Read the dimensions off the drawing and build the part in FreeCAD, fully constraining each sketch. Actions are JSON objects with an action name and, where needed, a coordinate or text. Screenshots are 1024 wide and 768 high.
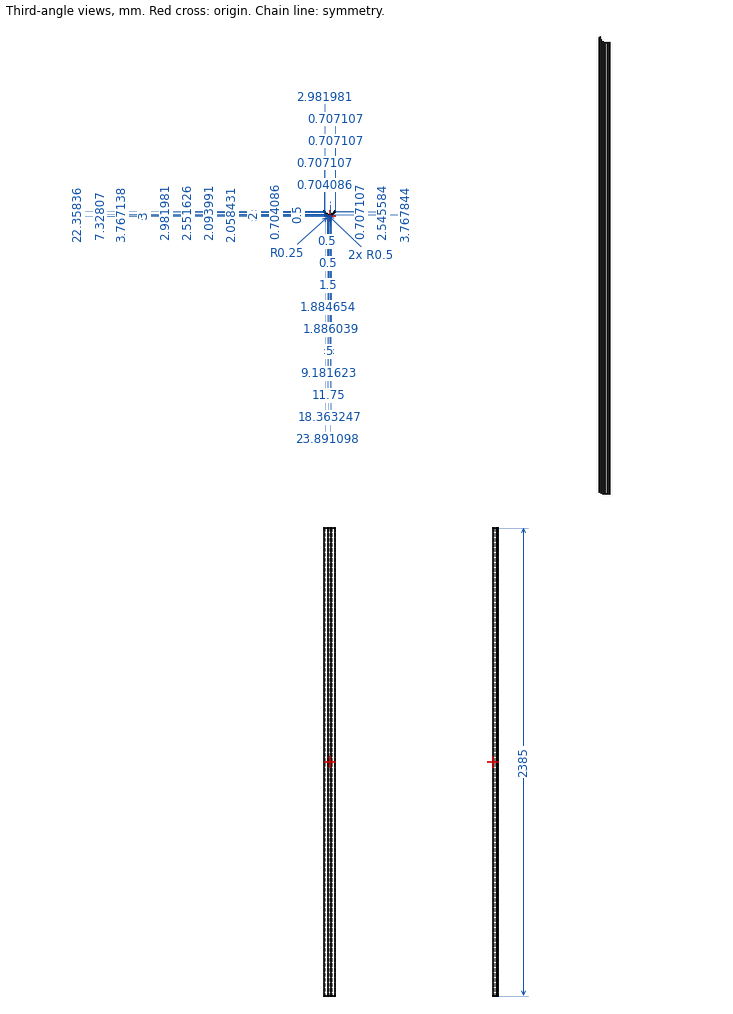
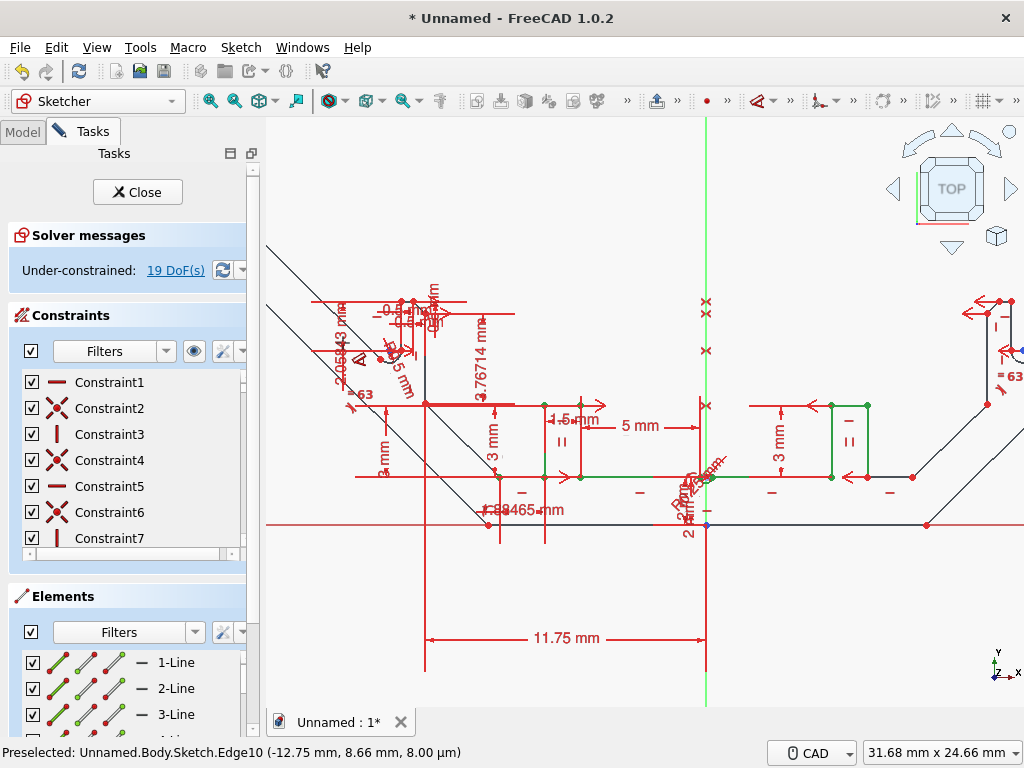
{"action": "scroll", "coordinate": [521, 478], "scroll_direction": "down", "scroll_amount": 6}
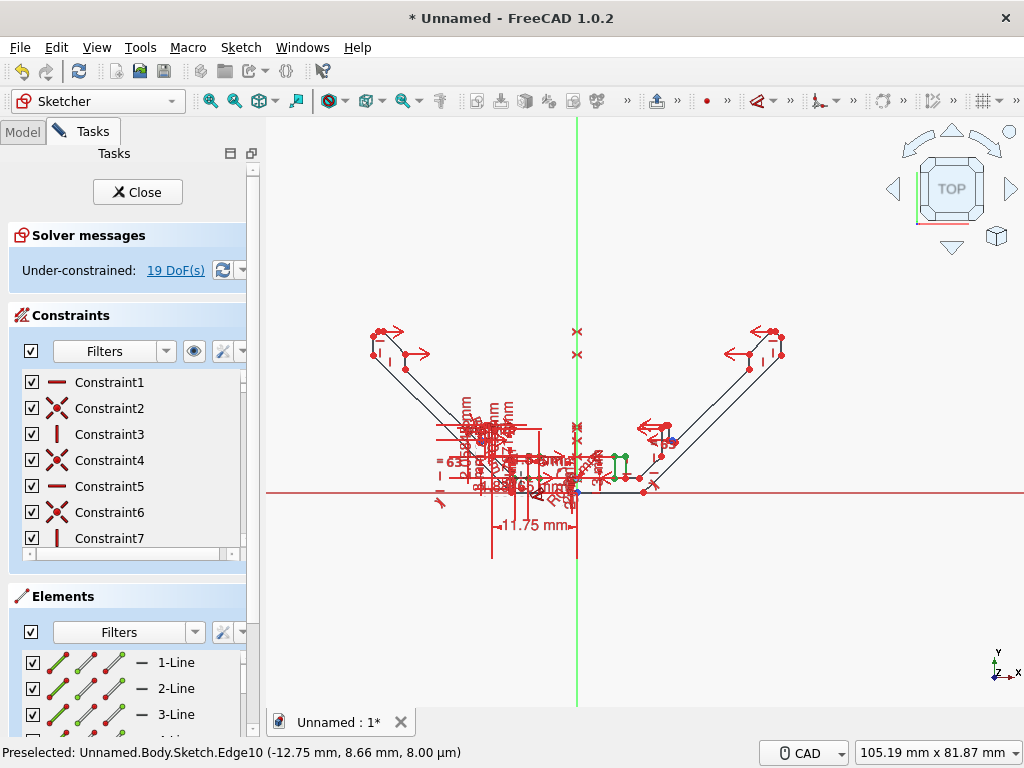
{"action": "scroll", "coordinate": [405, 365], "scroll_direction": "up", "scroll_amount": 6}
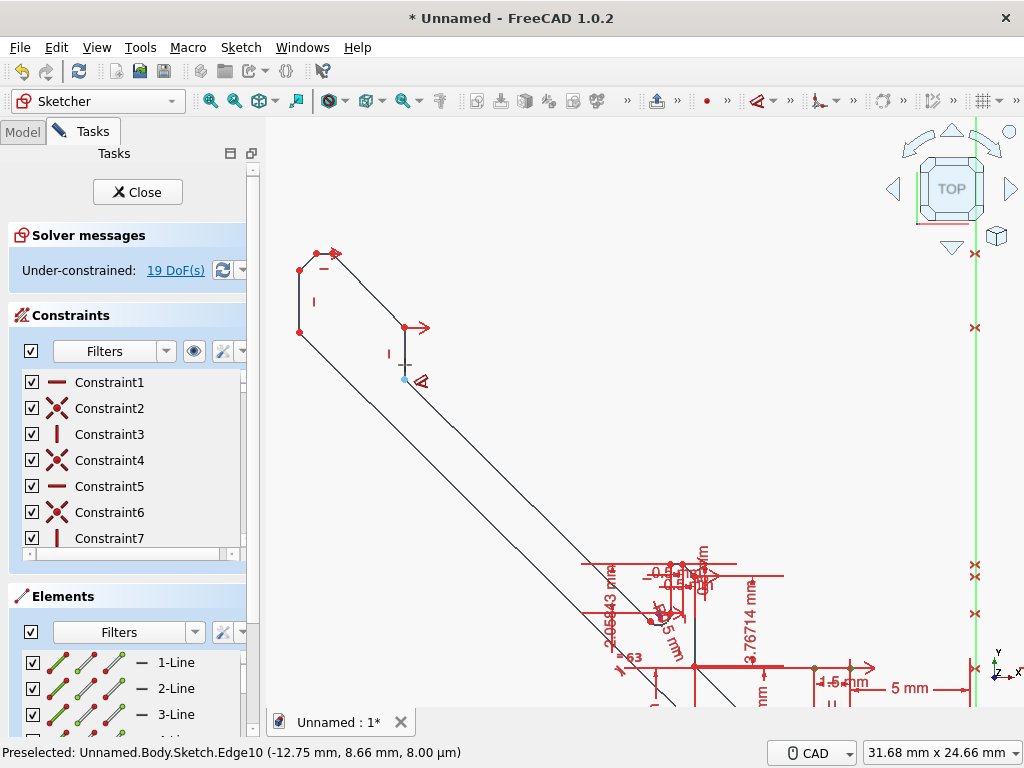
{"action": "left_click", "coordinate": [405, 364]}
{"action": "left_click", "coordinate": [371, 354]}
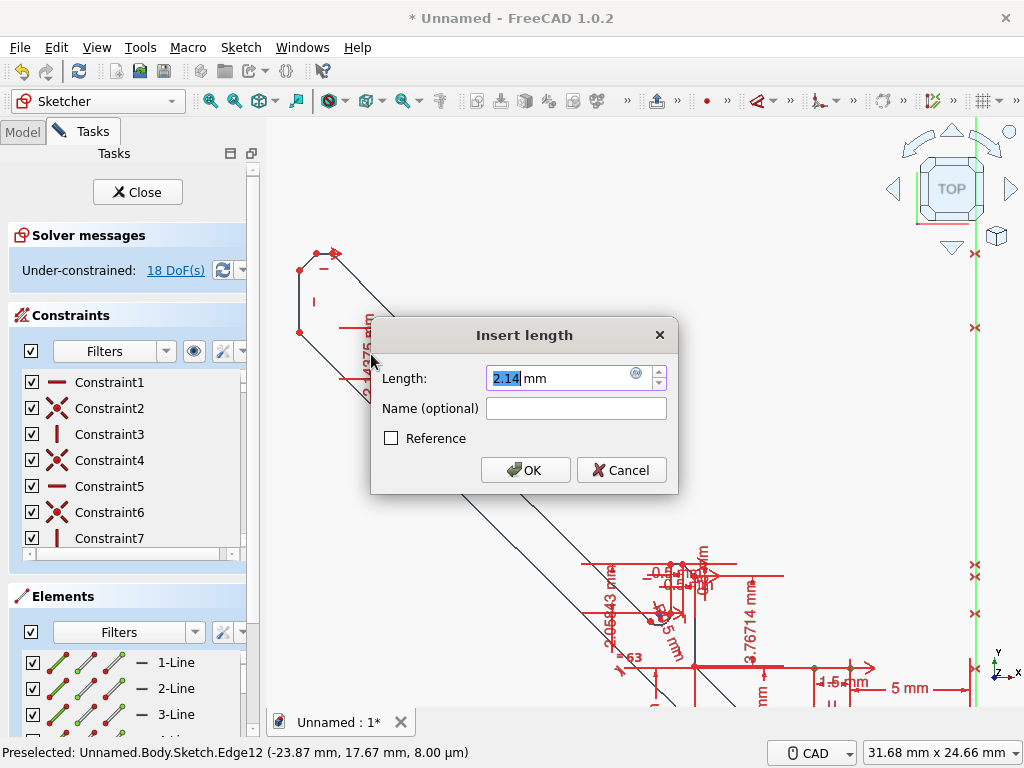
{"action": "type", "text": "2.093991"}
{"action": "key", "text": "Return"}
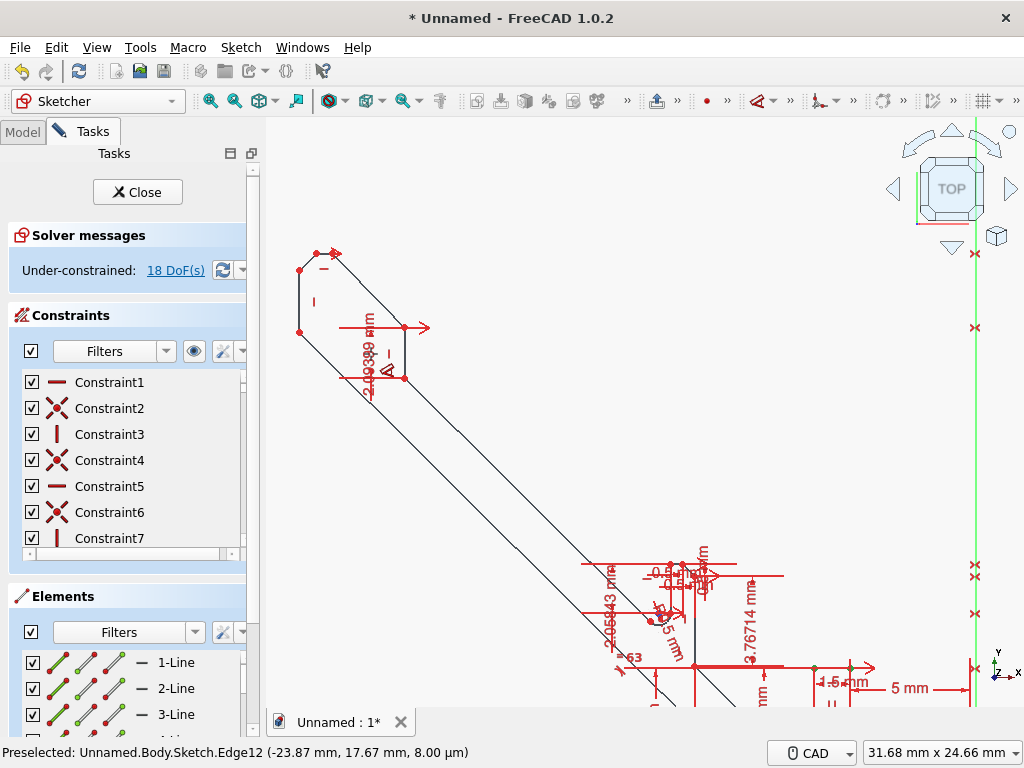
{"action": "scroll", "coordinate": [324, 254], "scroll_direction": "up", "scroll_amount": 5}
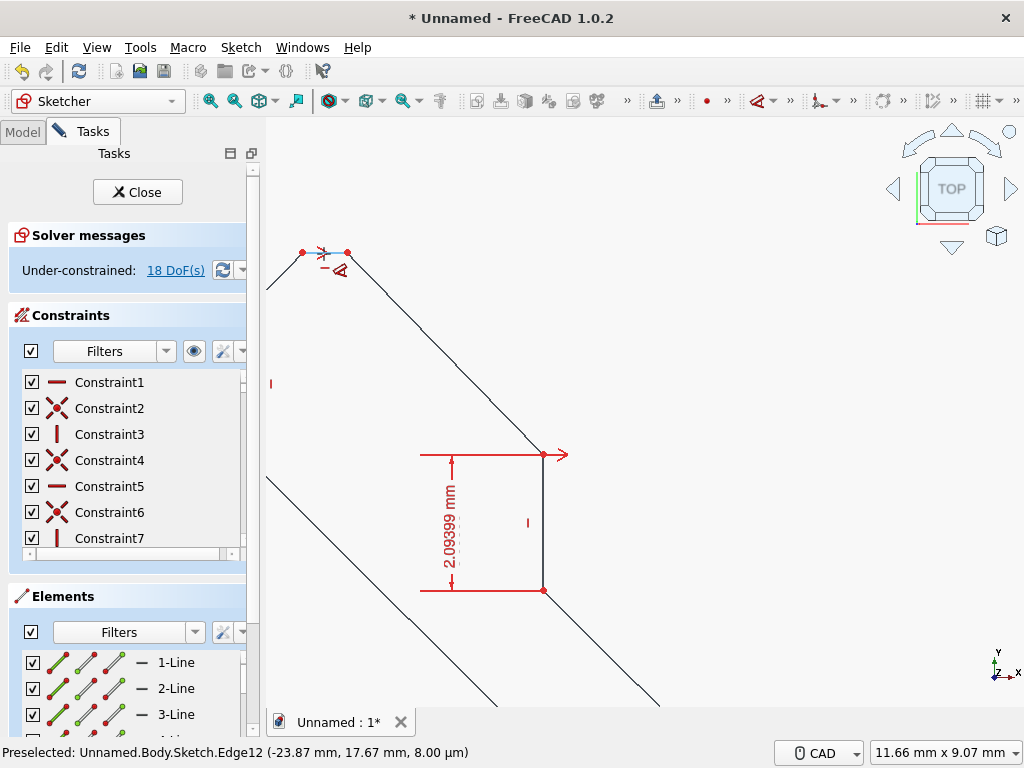
{"action": "left_click", "coordinate": [325, 253]}
{"action": "left_click", "coordinate": [325, 219]}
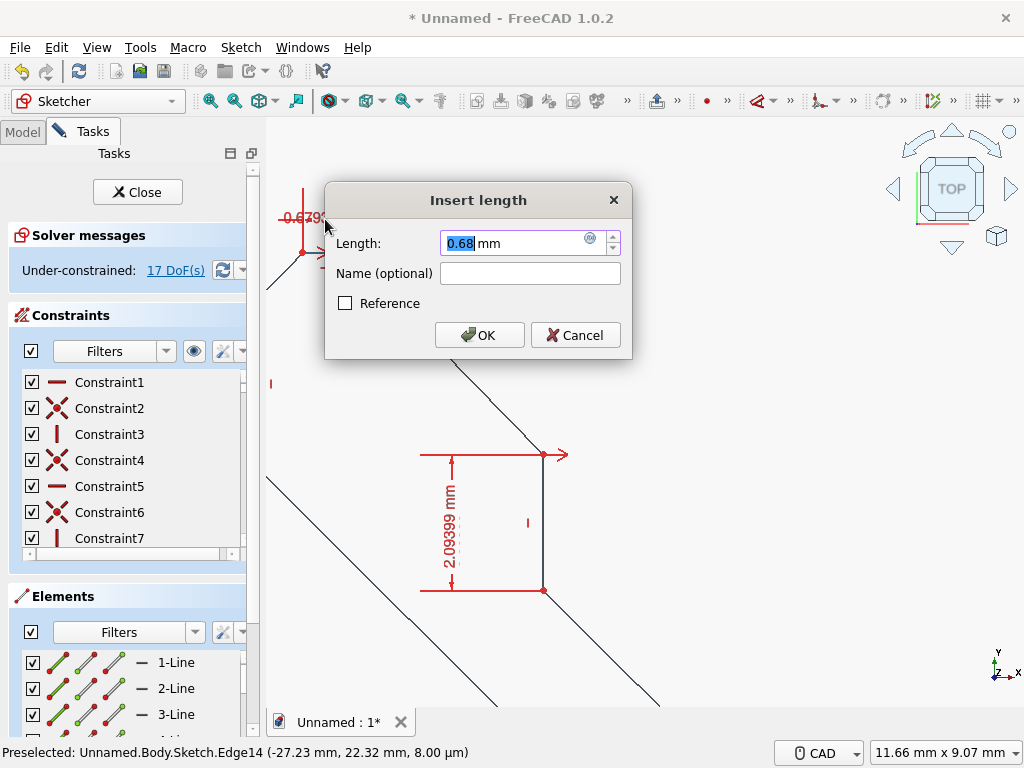
{"action": "type", "text": "0.707107"}
{"action": "key", "text": "Return"}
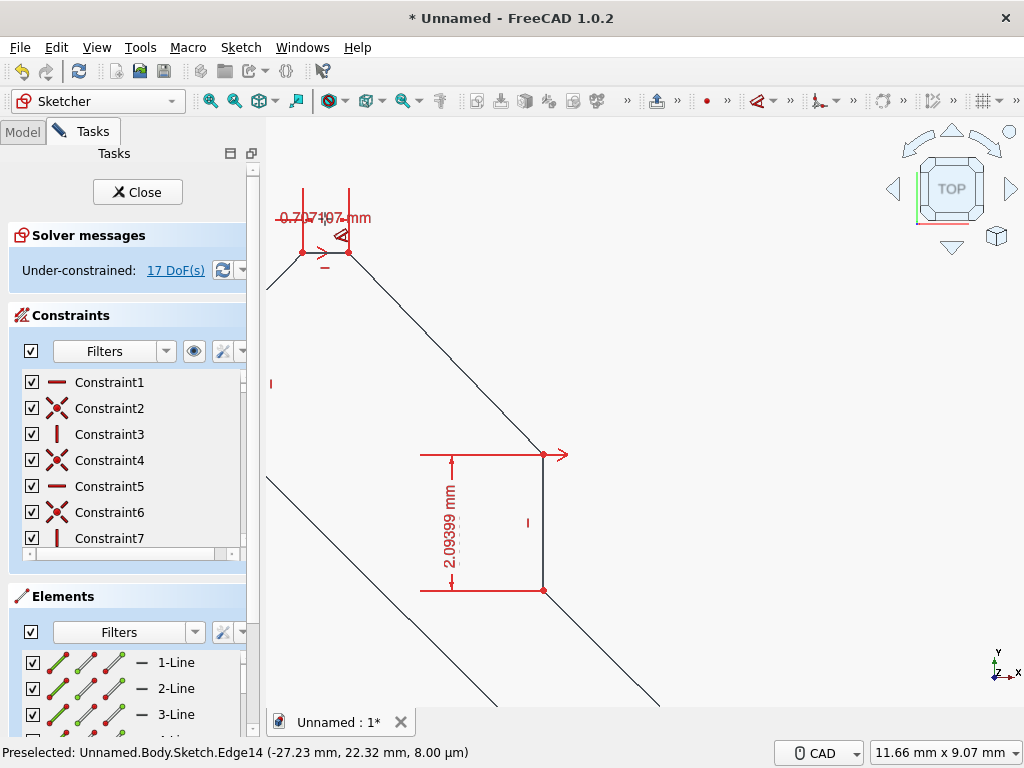
{"action": "scroll", "coordinate": [387, 341], "scroll_direction": "down", "scroll_amount": 11}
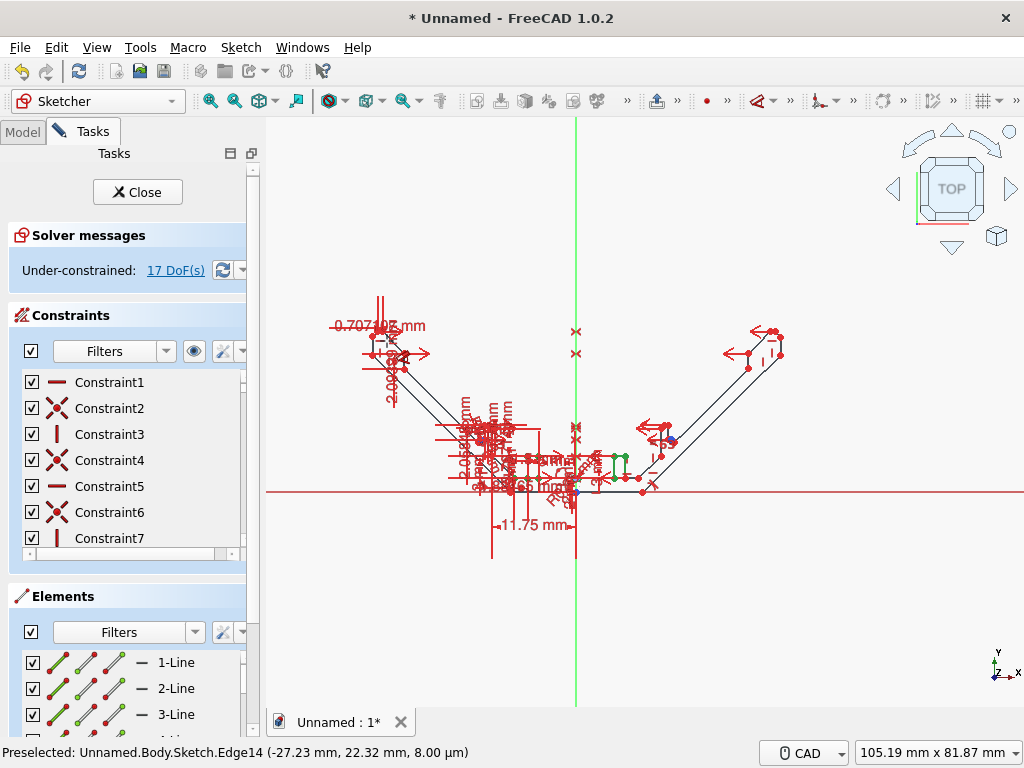
{"action": "scroll", "coordinate": [373, 342], "scroll_direction": "up", "scroll_amount": 5}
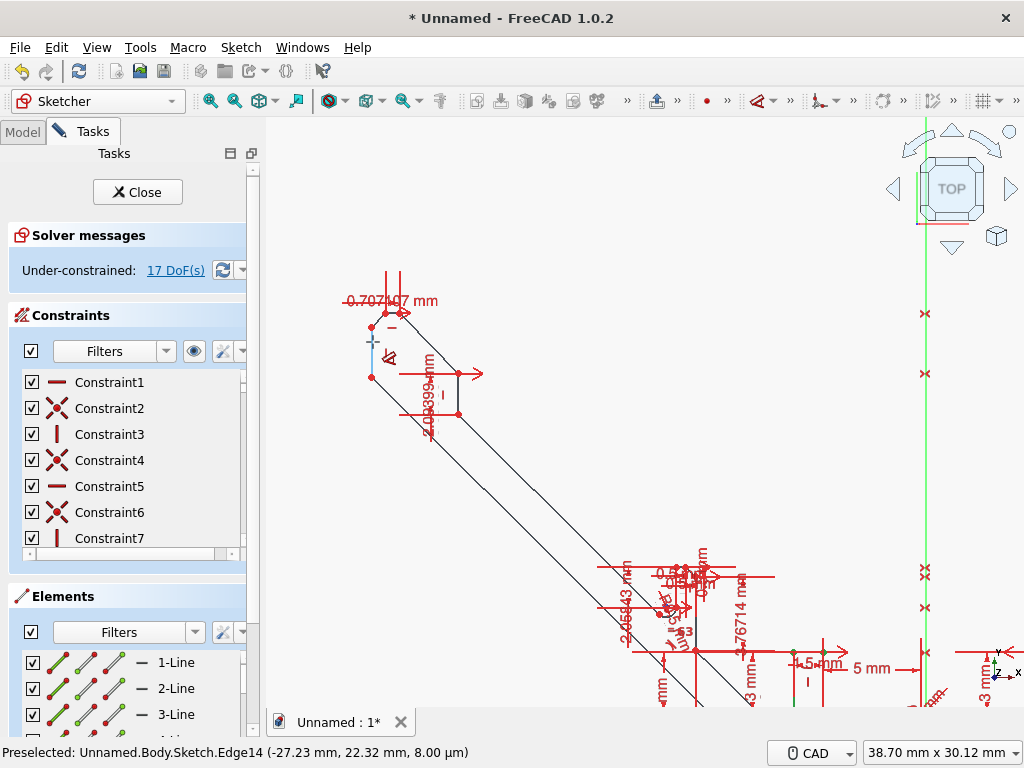
{"action": "left_click", "coordinate": [372, 342]}
{"action": "left_click", "coordinate": [338, 352]}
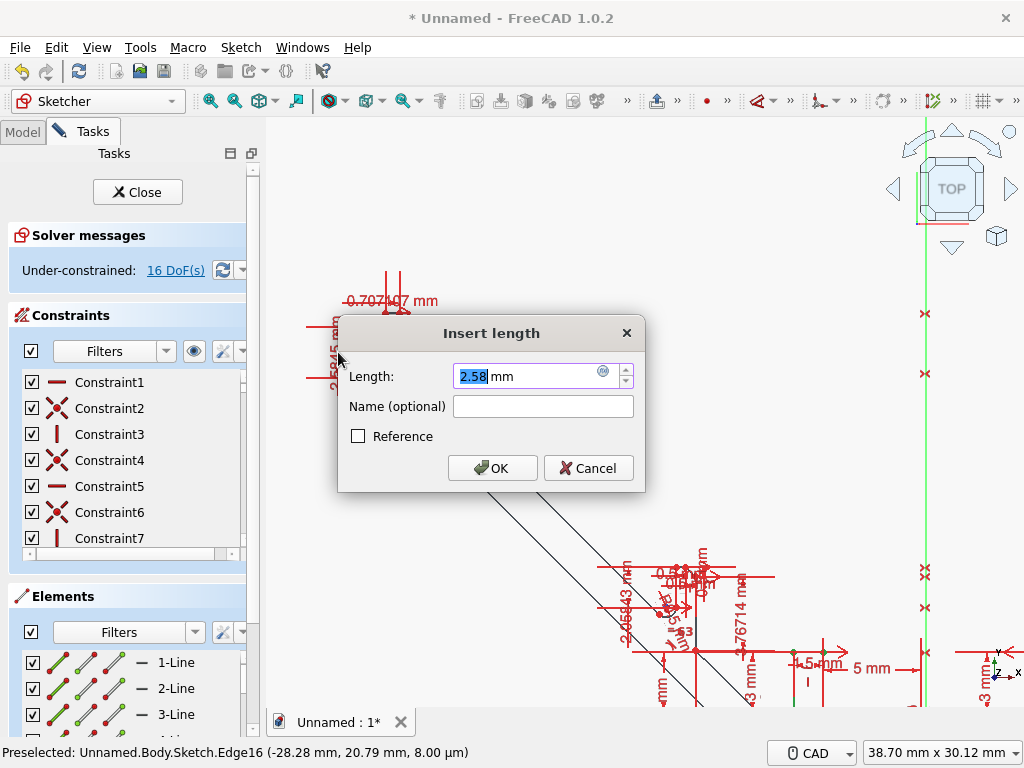
{"action": "type", "text": "2.551626"}
{"action": "key", "text": "Return"}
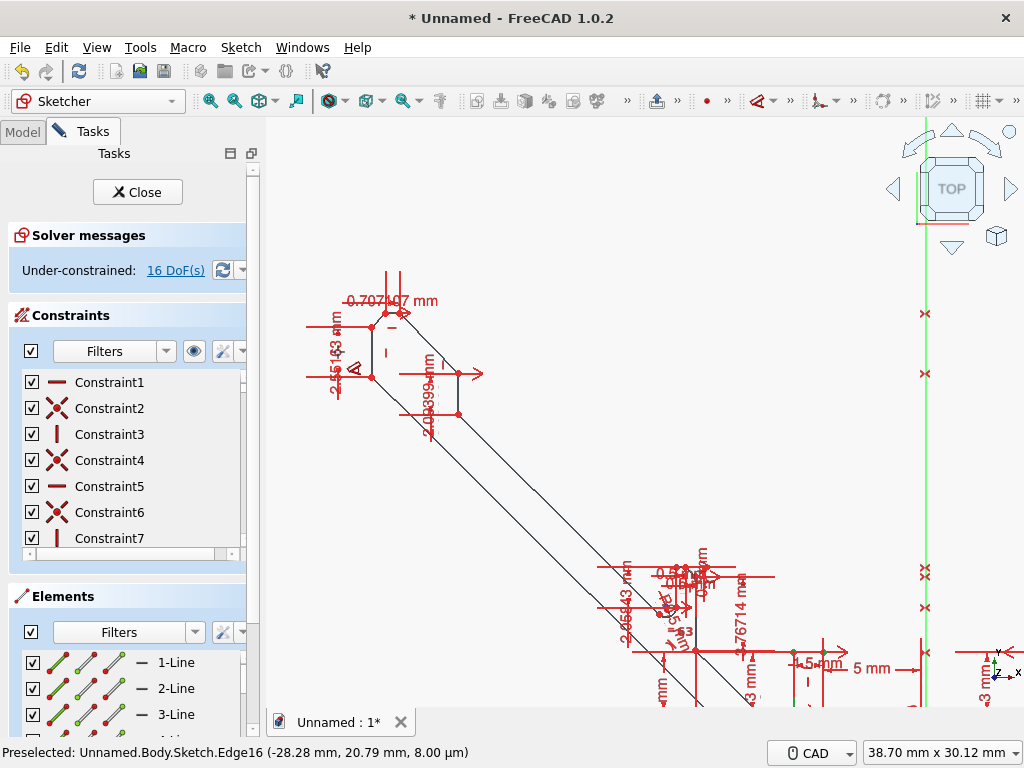
{"action": "scroll", "coordinate": [373, 343], "scroll_direction": "down", "scroll_amount": 5}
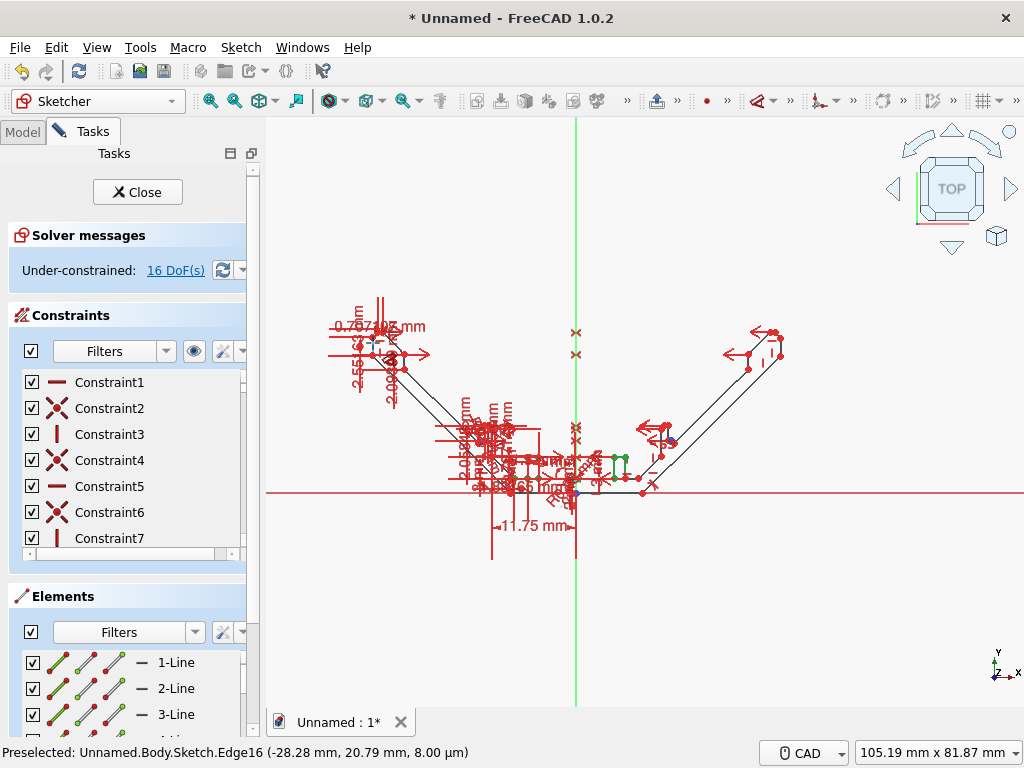
{"action": "scroll", "coordinate": [781, 351], "scroll_direction": "up", "scroll_amount": 5}